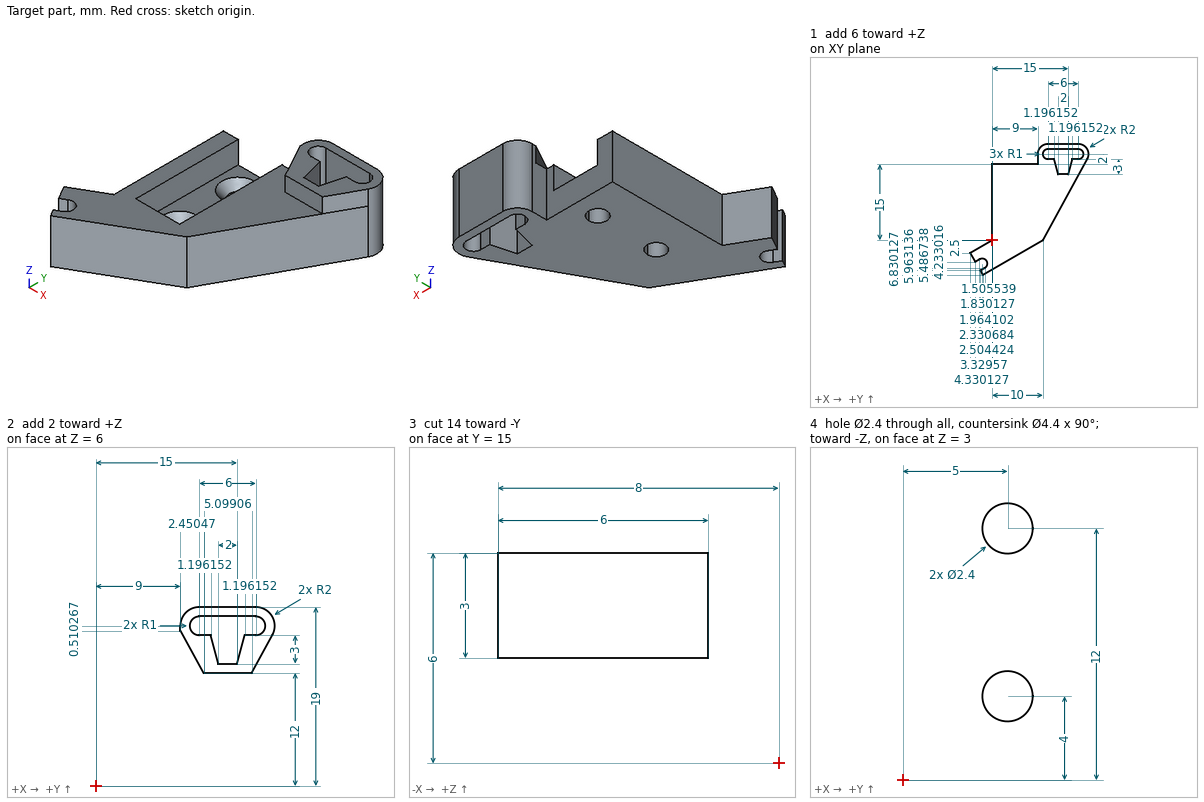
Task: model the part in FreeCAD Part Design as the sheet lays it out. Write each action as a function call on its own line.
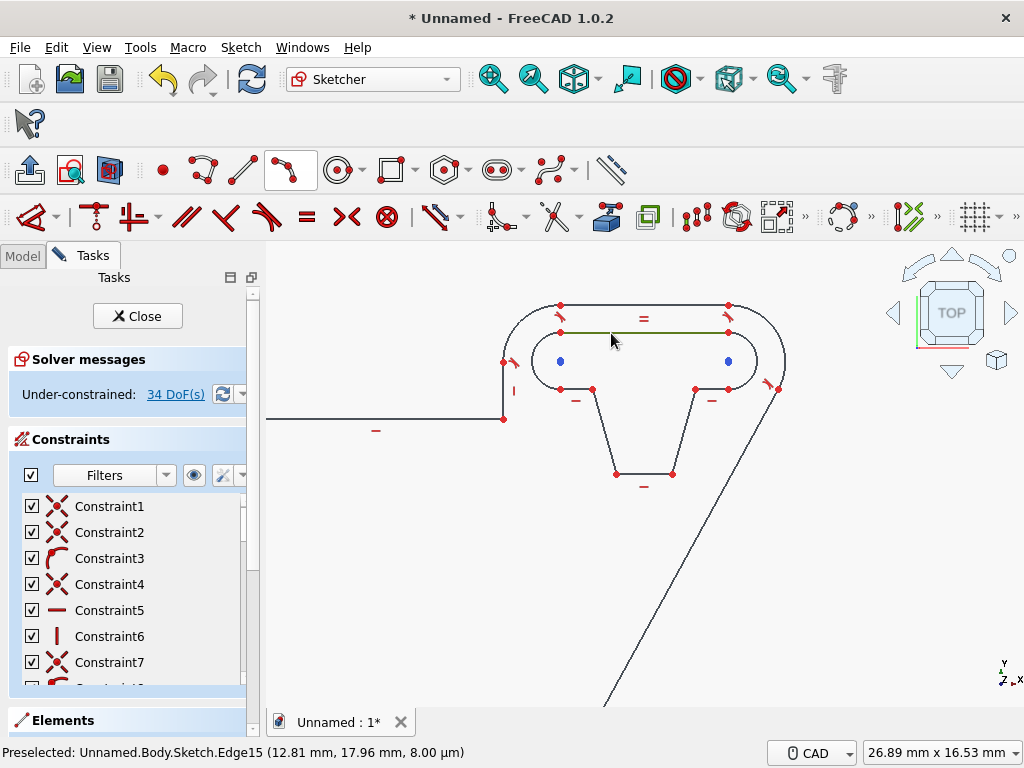
click(752, 378)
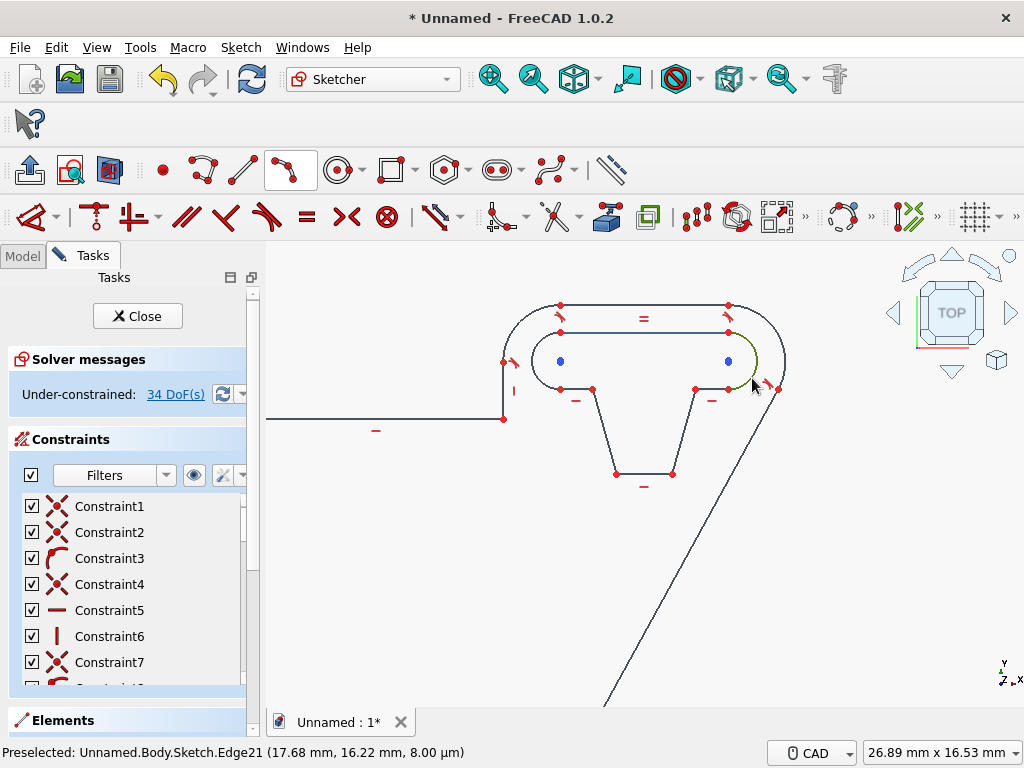
key(t)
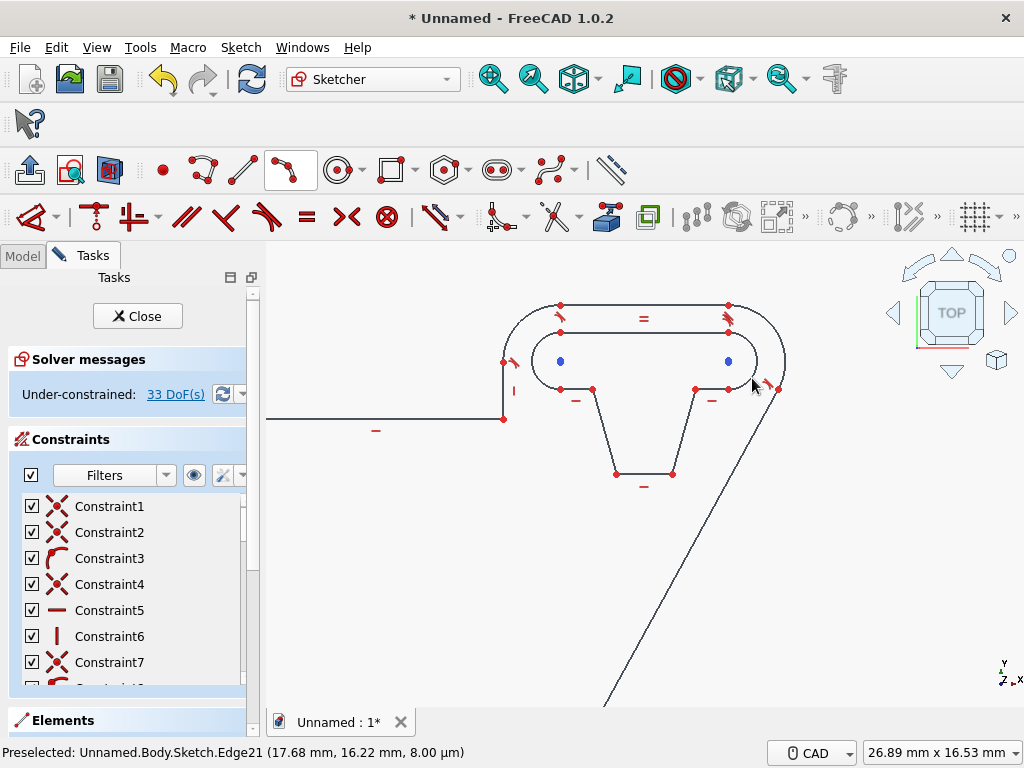
click(611, 333)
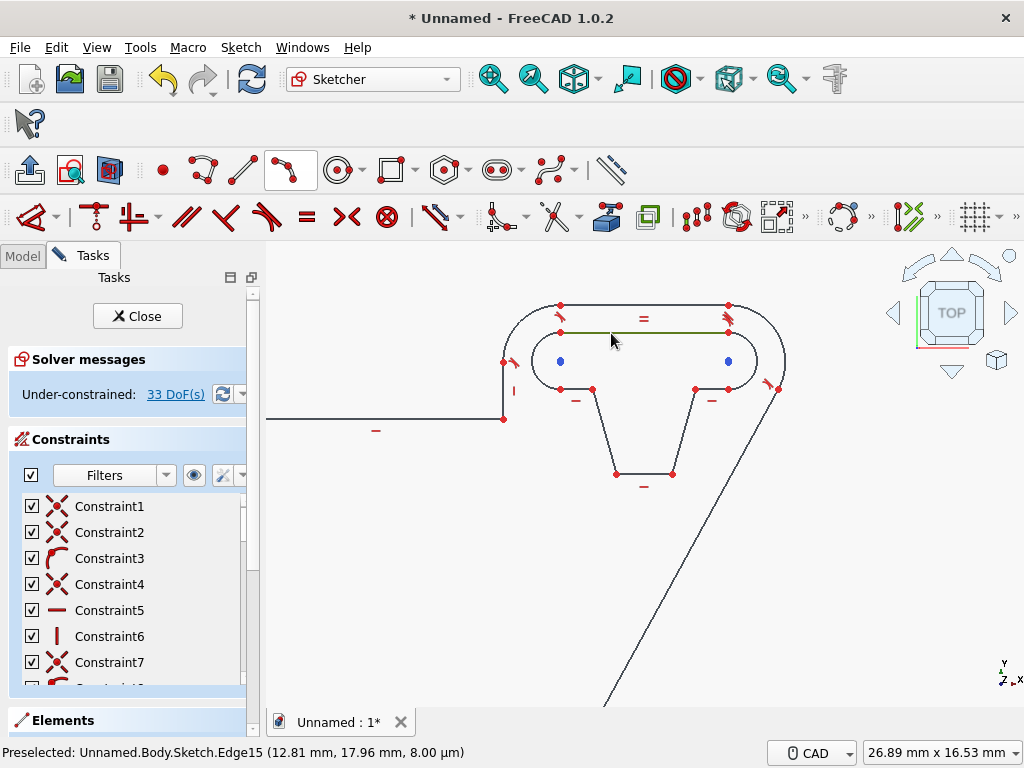
click(537, 344)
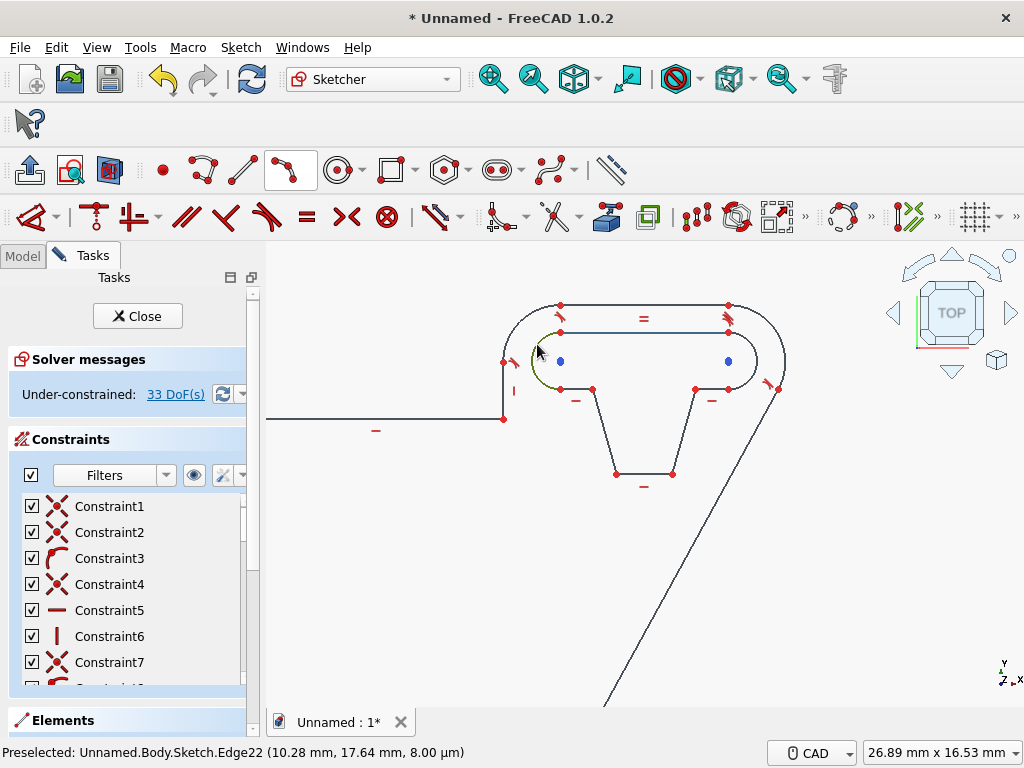
key(t)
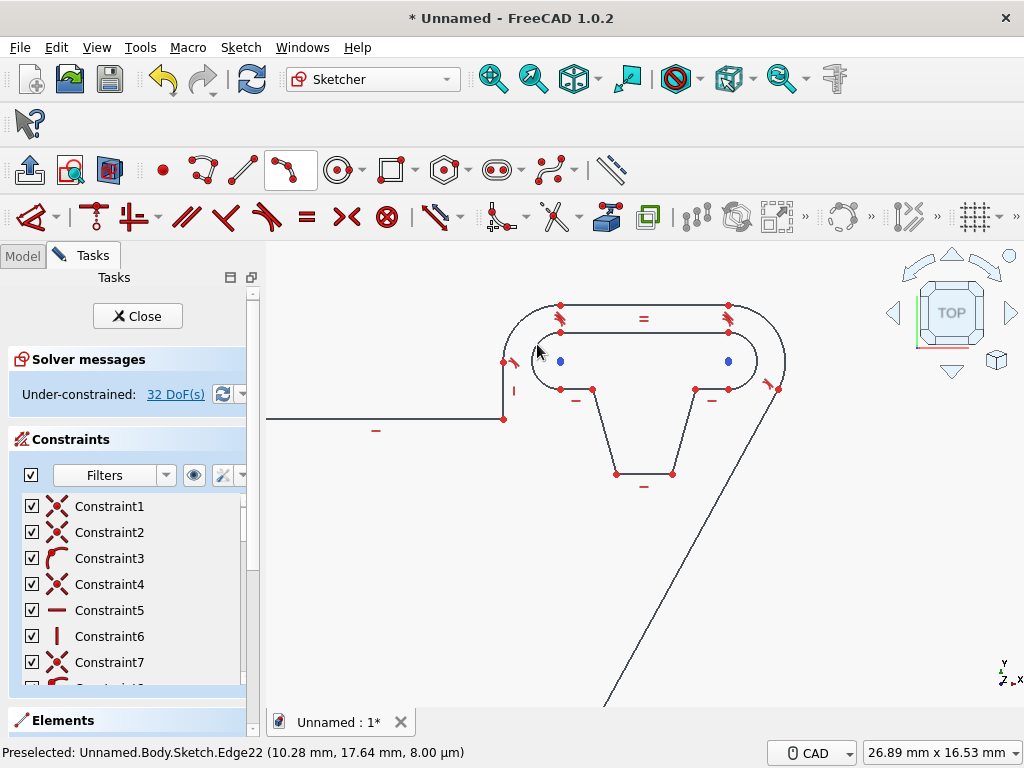
scroll(719, 389, up, 2)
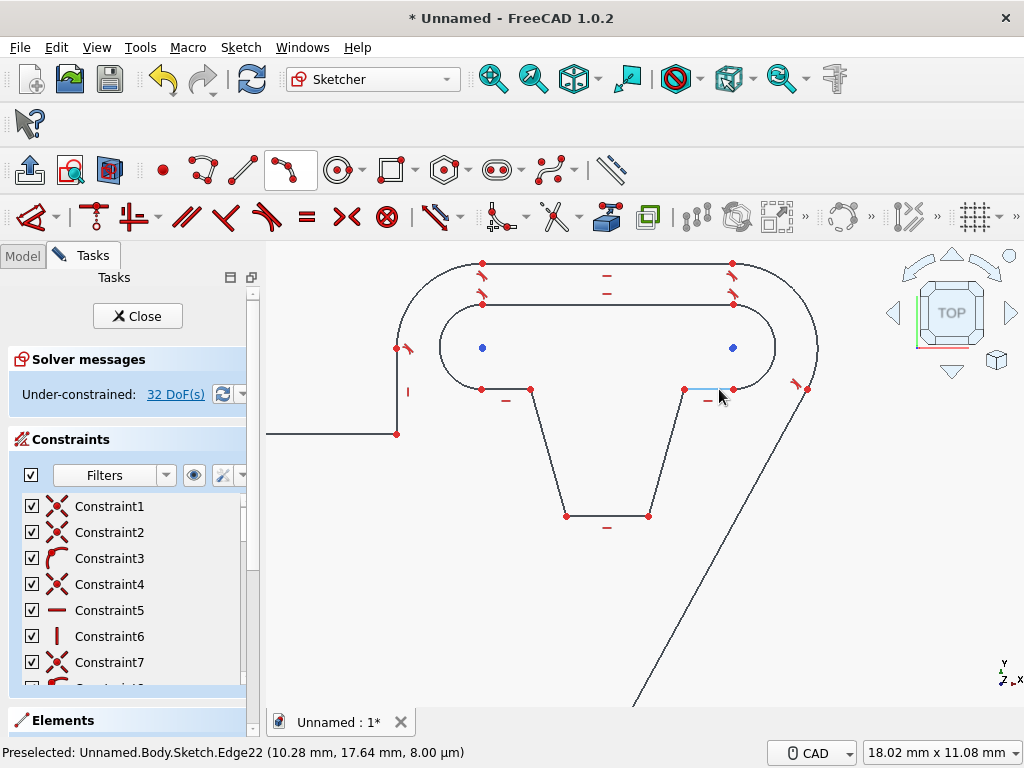
click(718, 389)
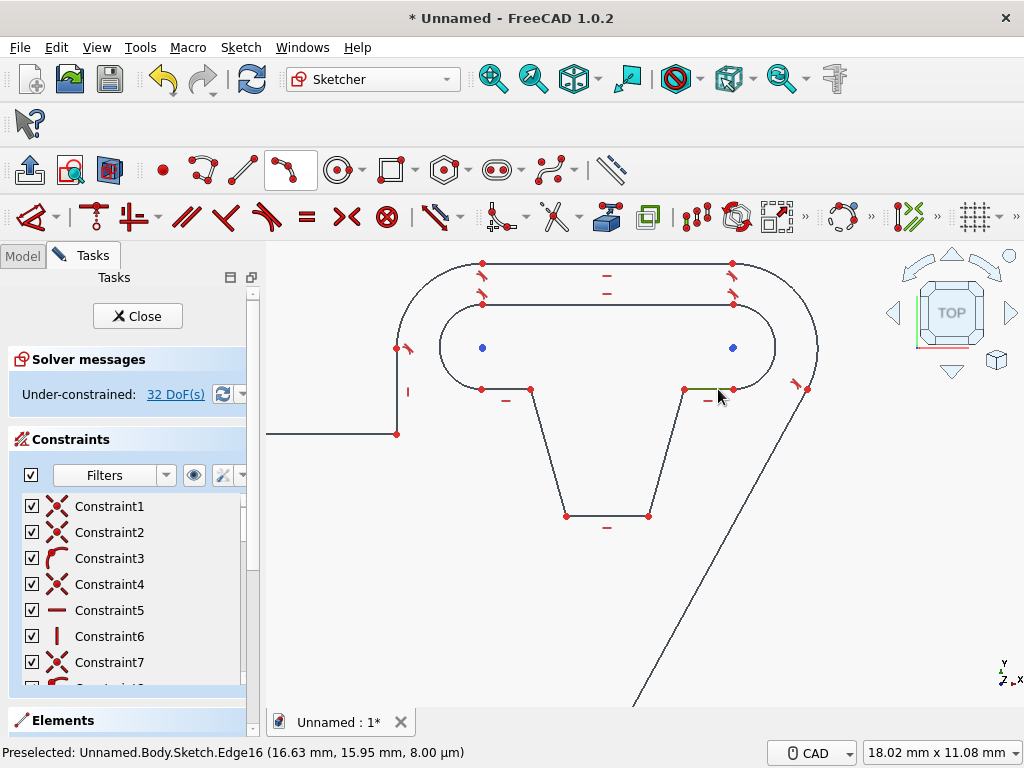
click(767, 372)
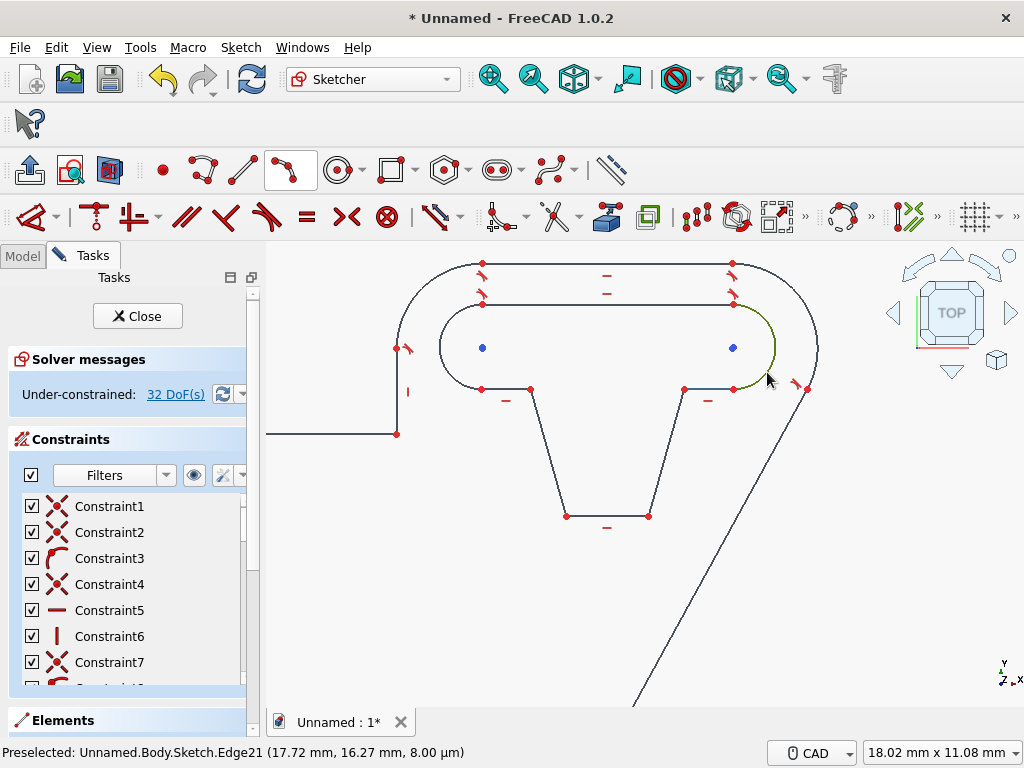
key(t)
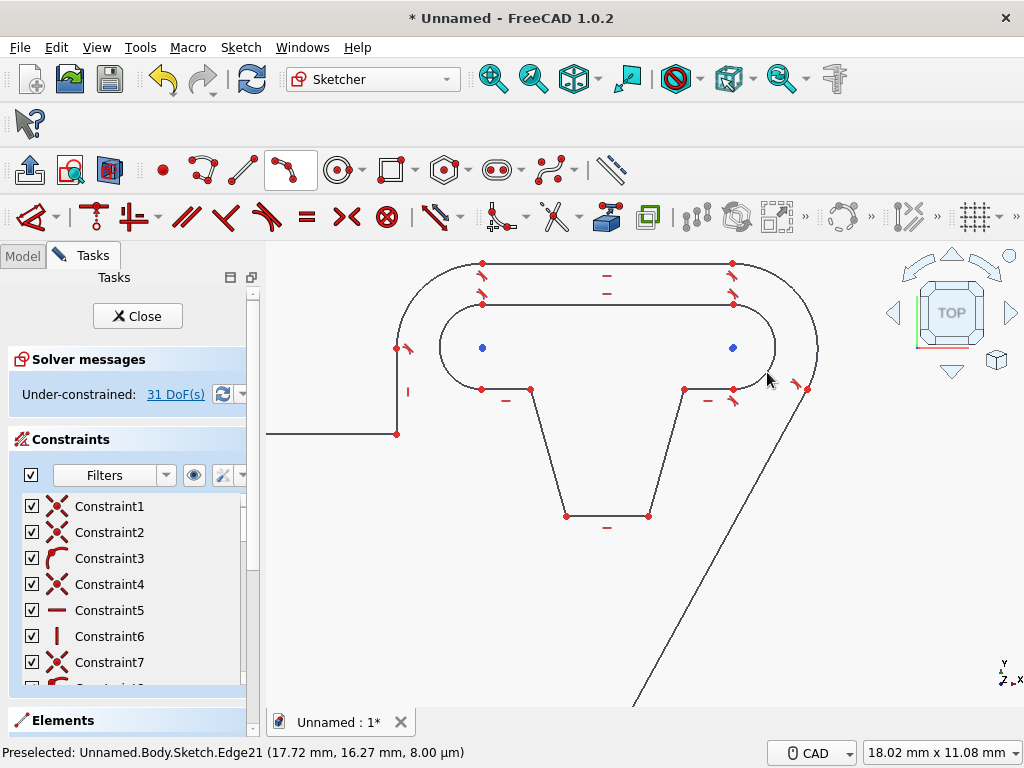
click(516, 389)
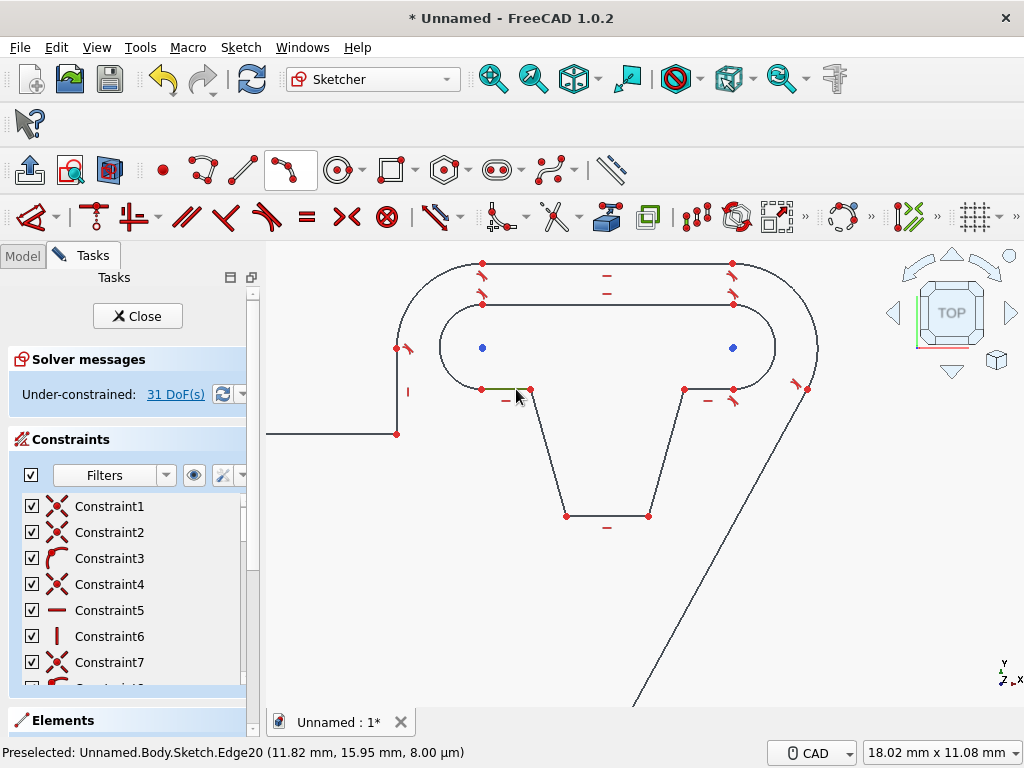
click(448, 322)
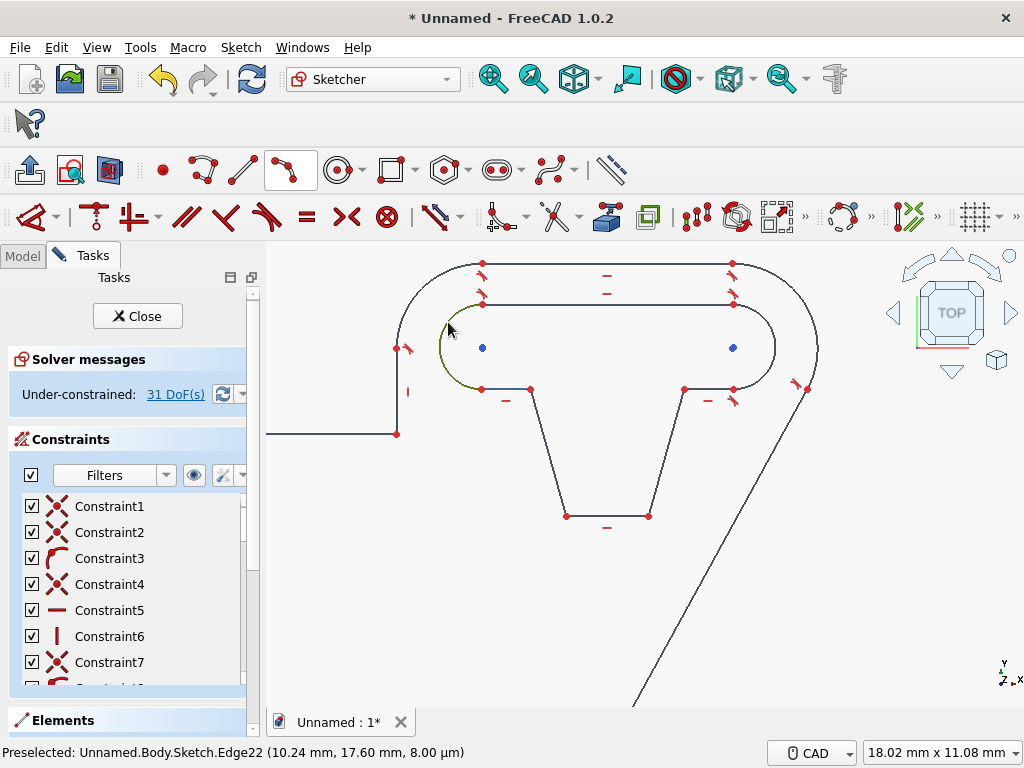
key(t)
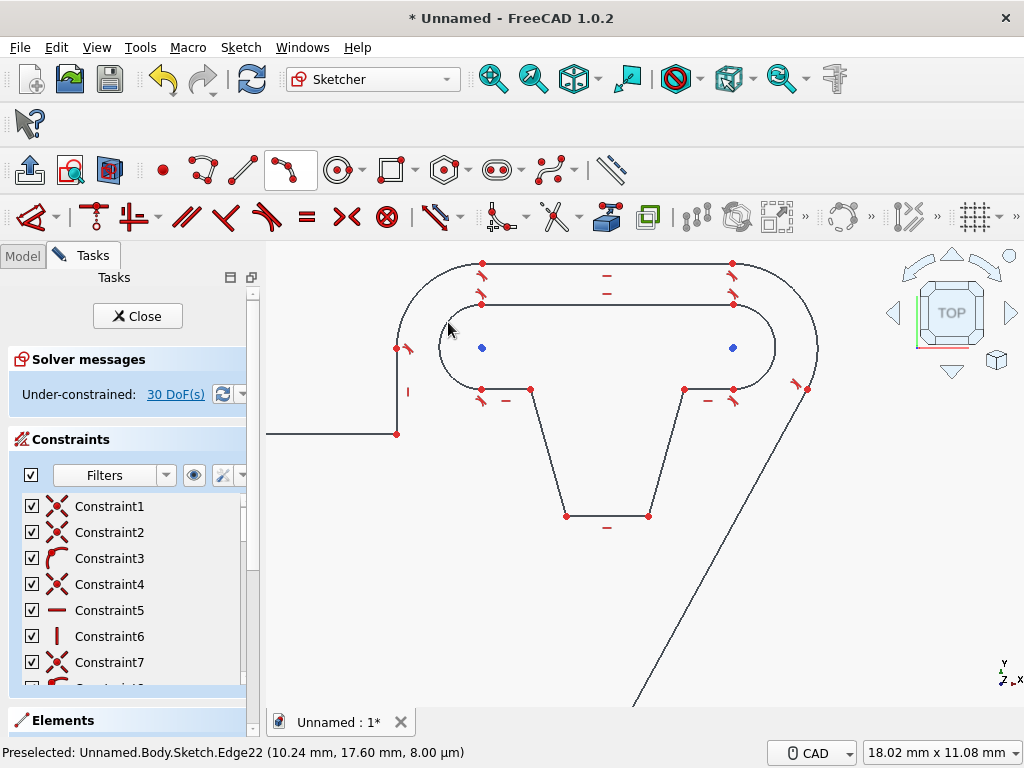
scroll(660, 366, down, 7)